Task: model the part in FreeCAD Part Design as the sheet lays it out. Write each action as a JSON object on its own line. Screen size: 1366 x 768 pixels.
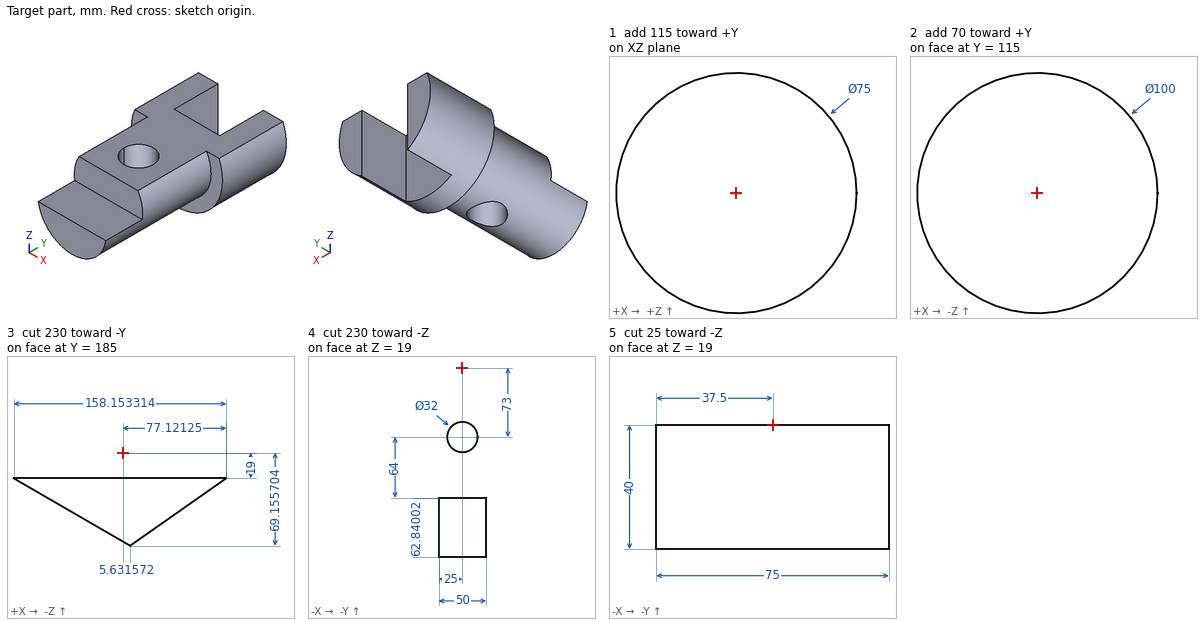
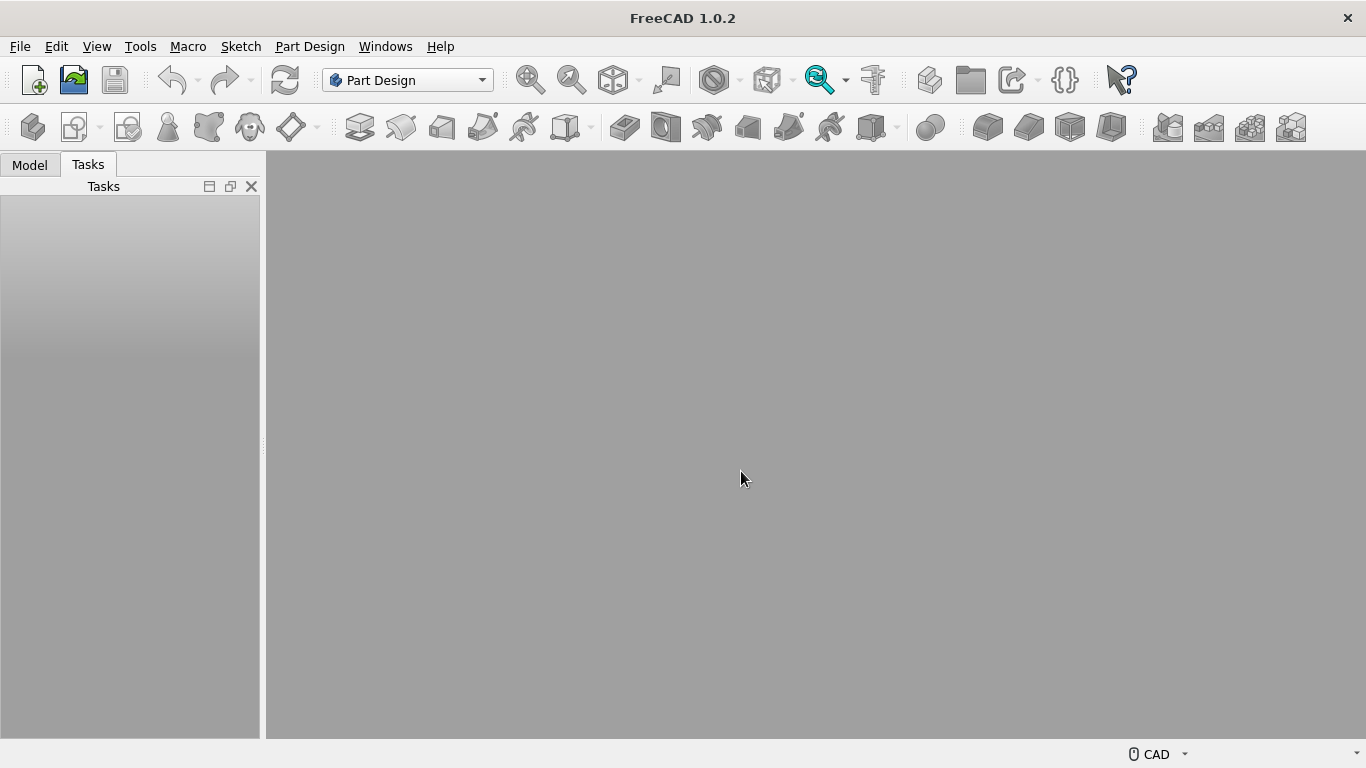
{"action": "left_click", "coordinate": [33, 80]}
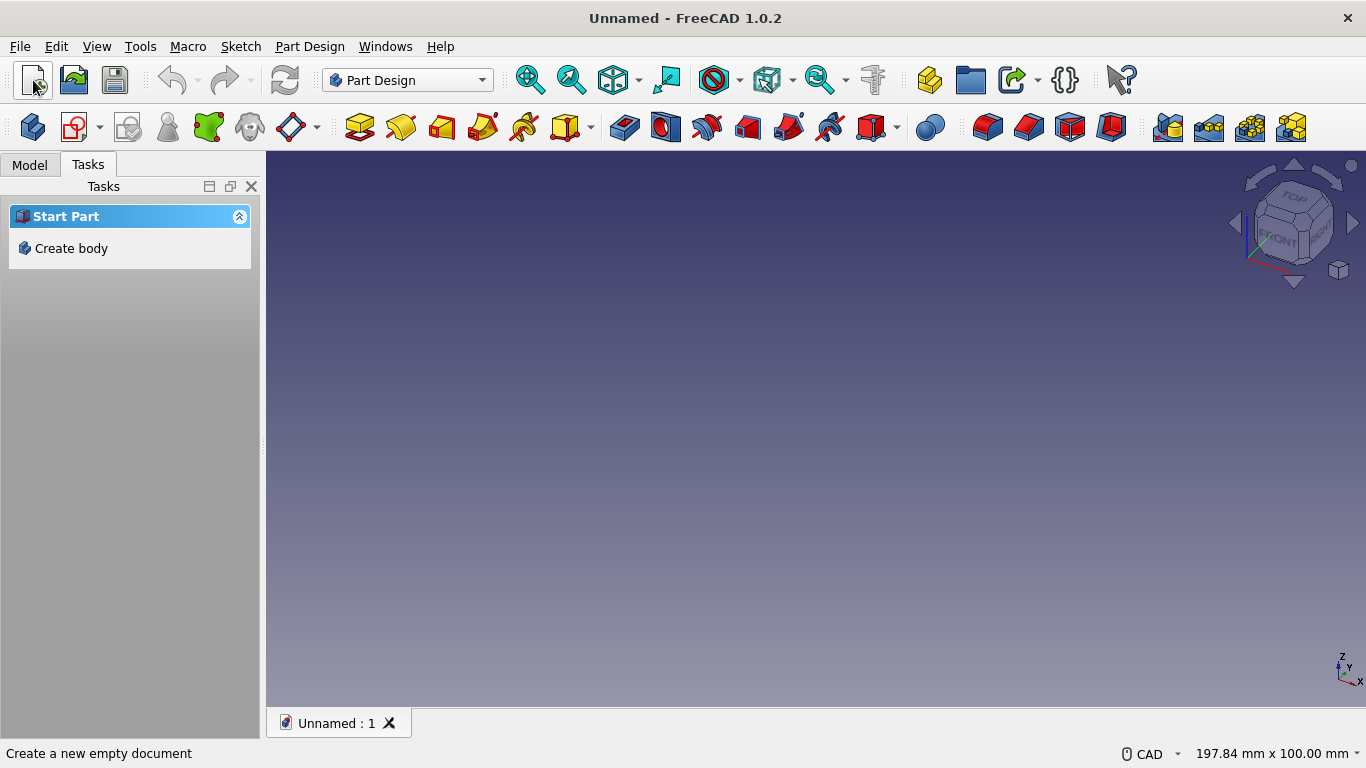
{"action": "left_click", "coordinate": [74, 128]}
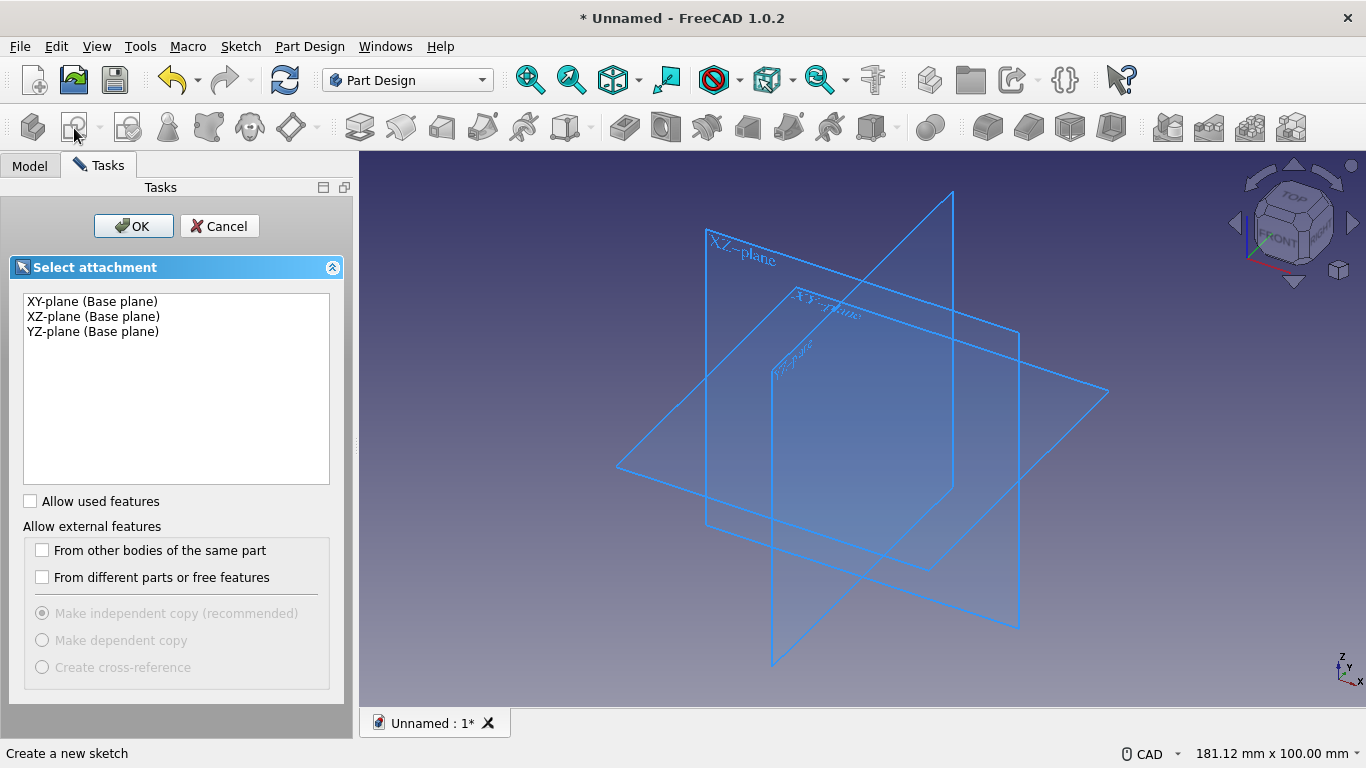
{"action": "left_click", "coordinate": [84, 316]}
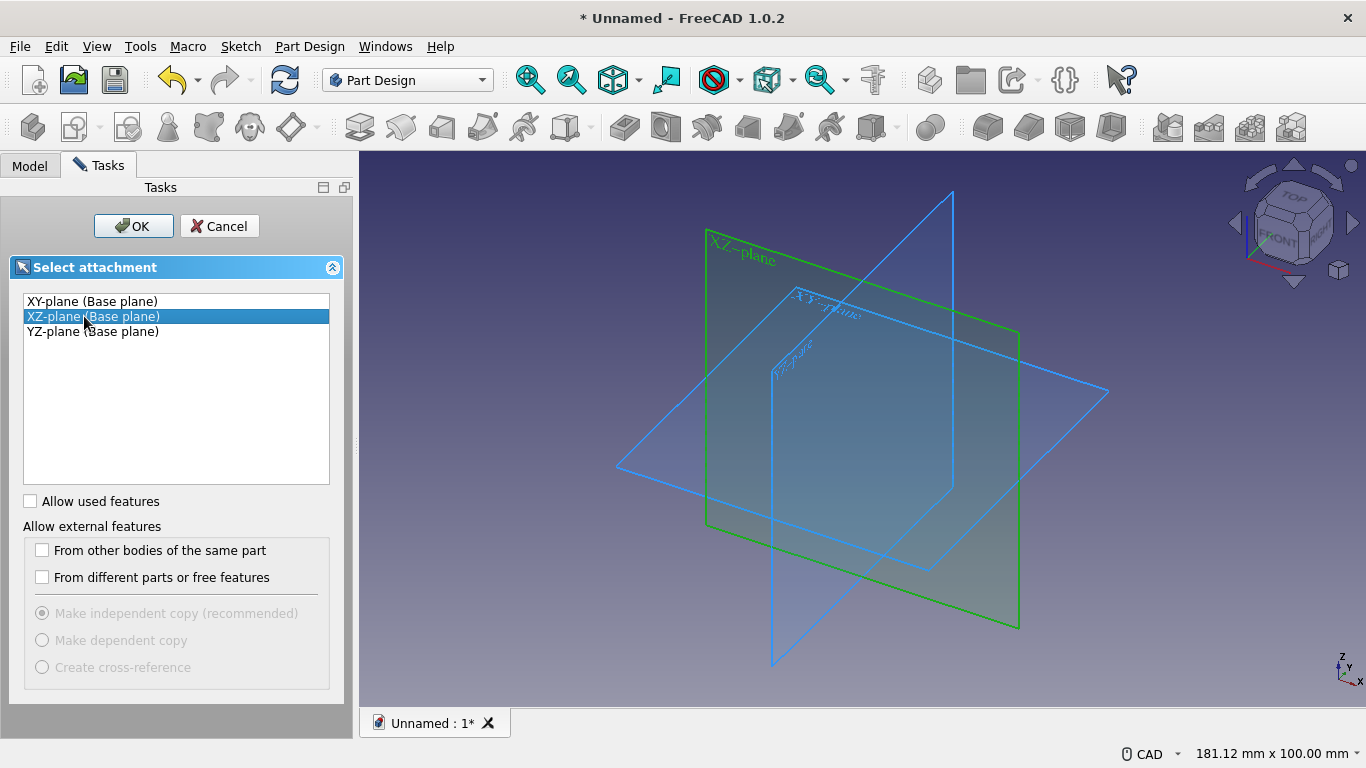
{"action": "left_click", "coordinate": [134, 226]}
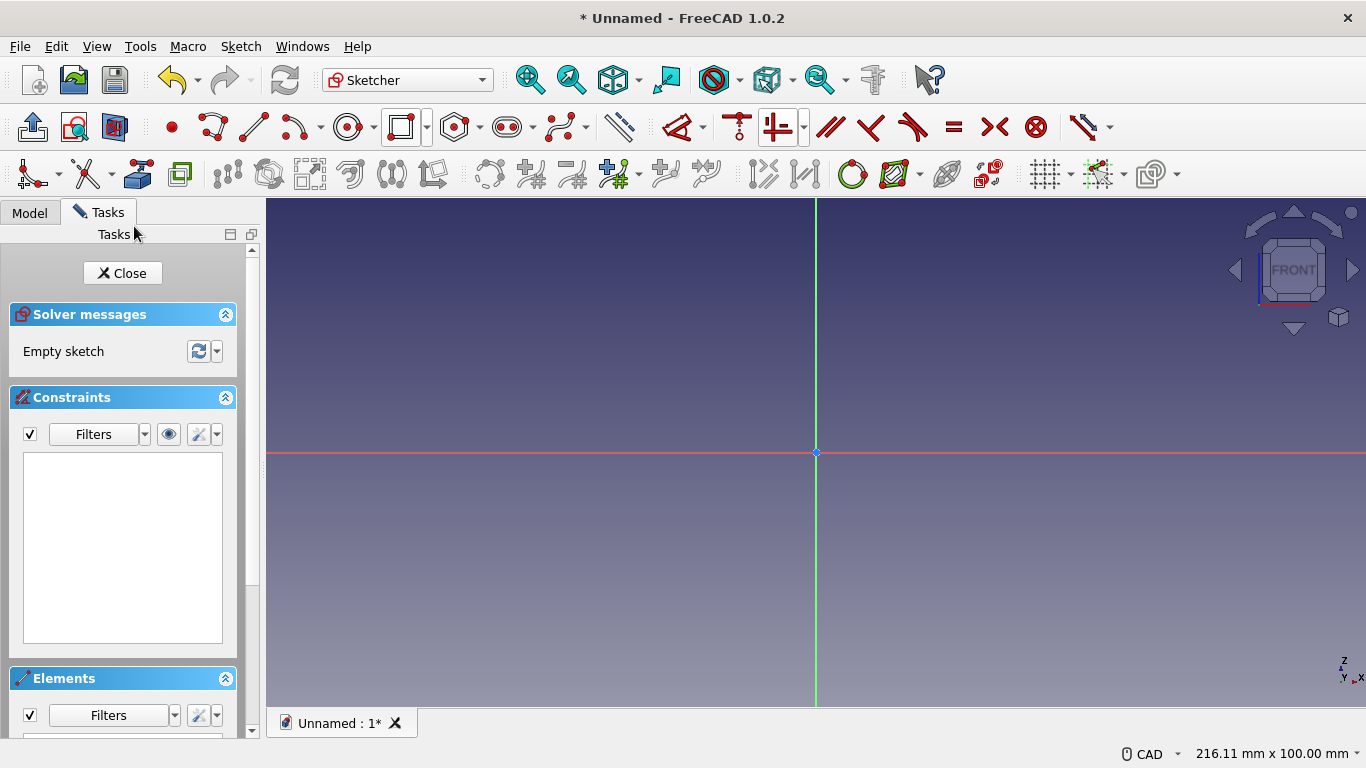
{"action": "left_click", "coordinate": [348, 128]}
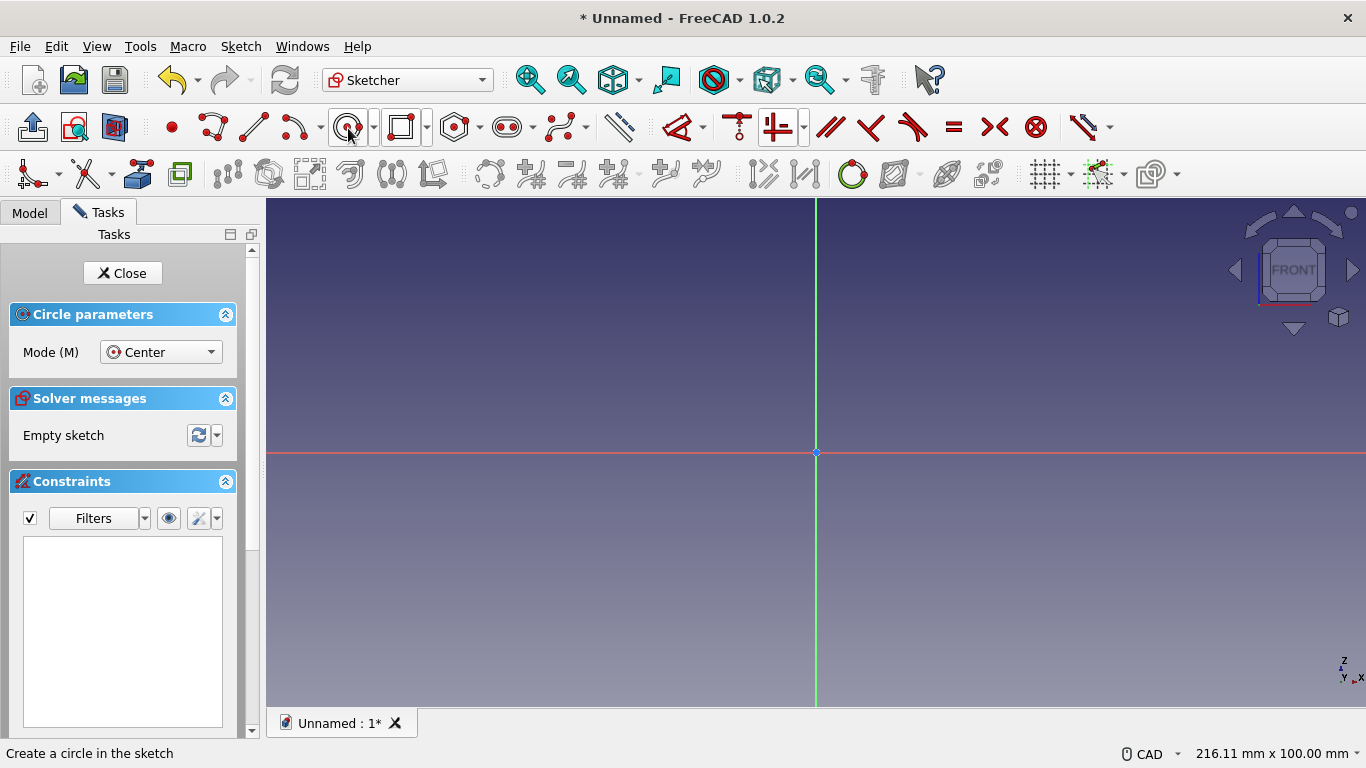
{"action": "left_click", "coordinate": [816, 452]}
{"action": "left_click", "coordinate": [951, 318]}
{"action": "key", "text": "Escape"}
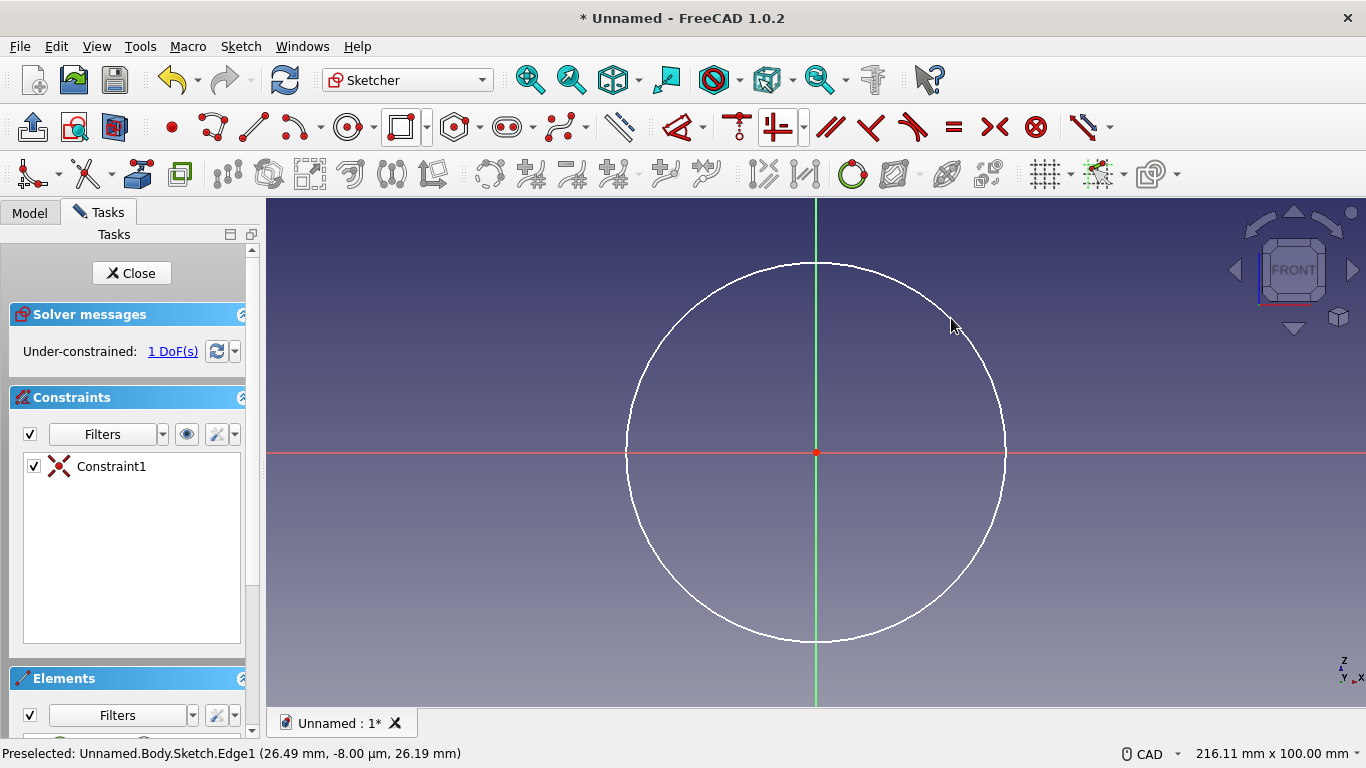
{"action": "left_click", "coordinate": [950, 318]}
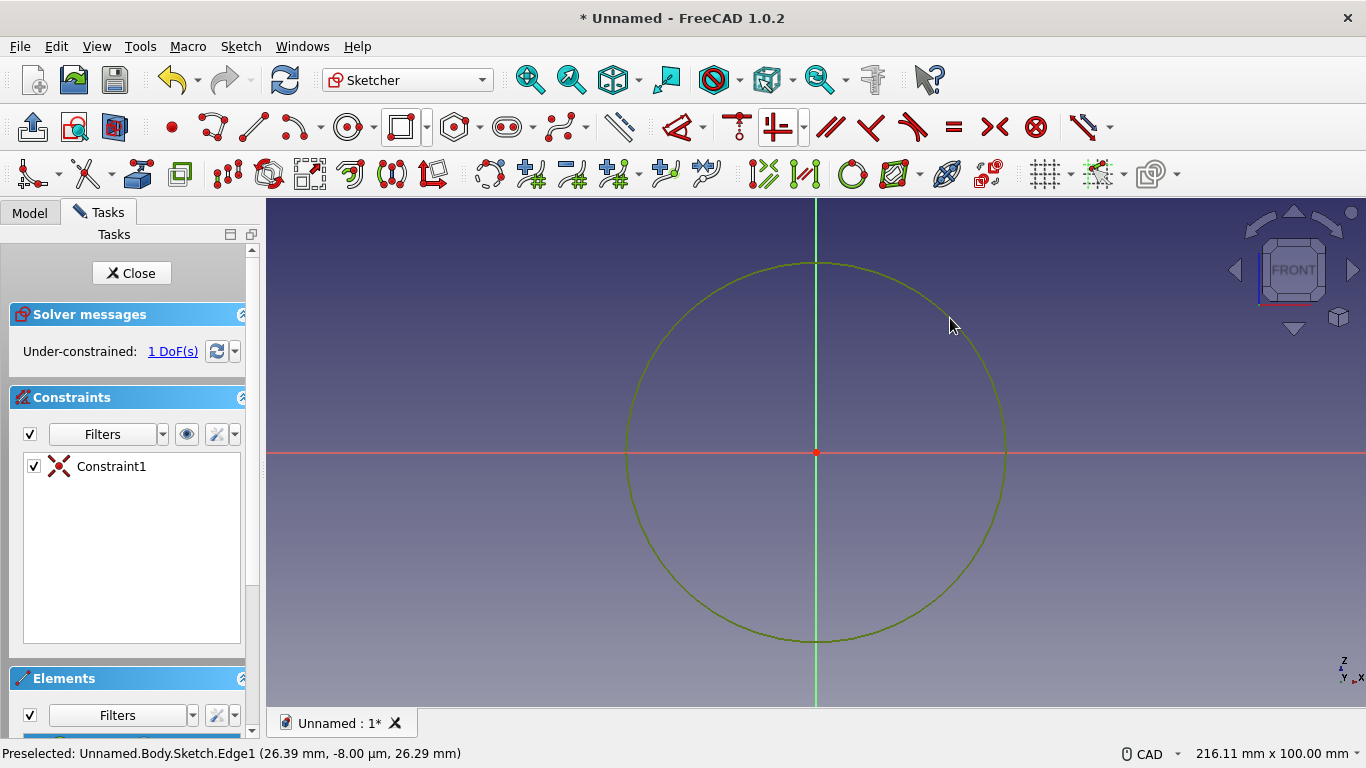
{"action": "left_click", "coordinate": [702, 128]}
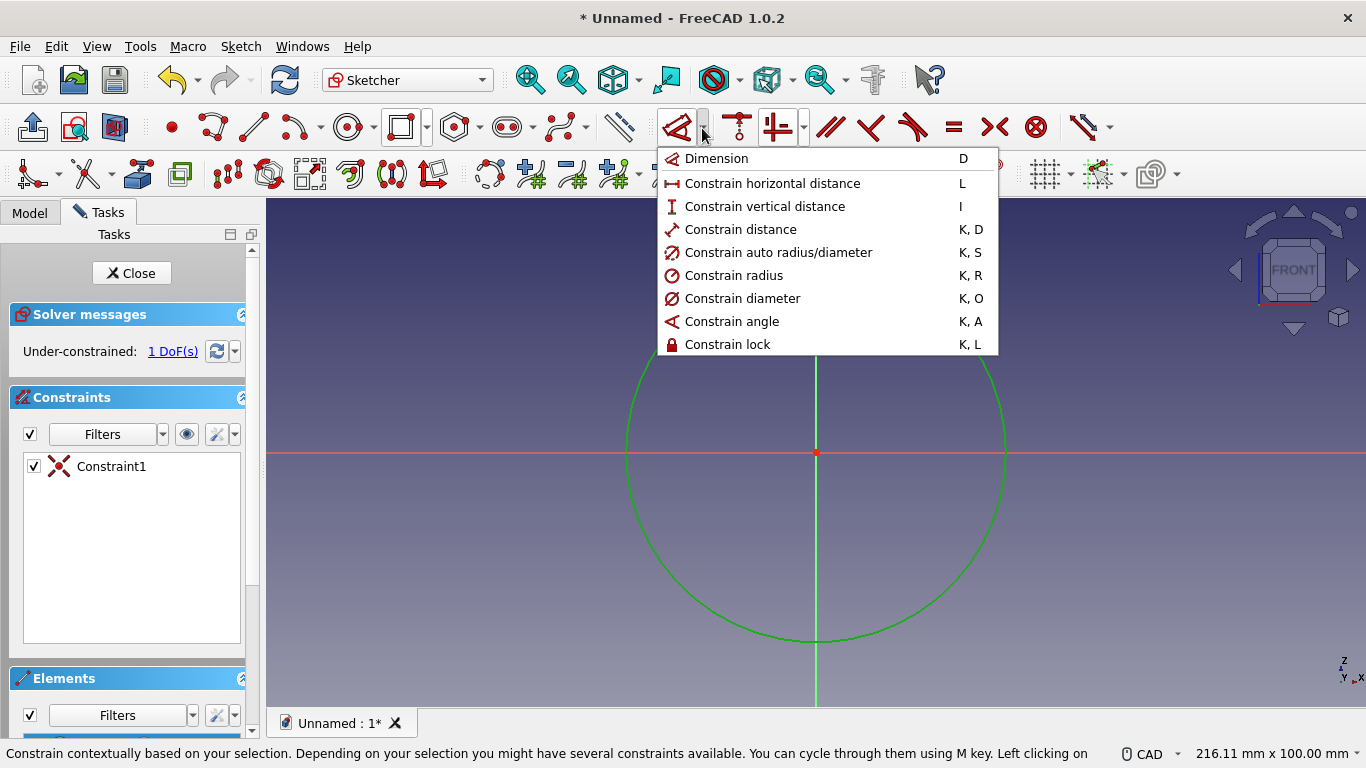
{"action": "left_click", "coordinate": [828, 298]}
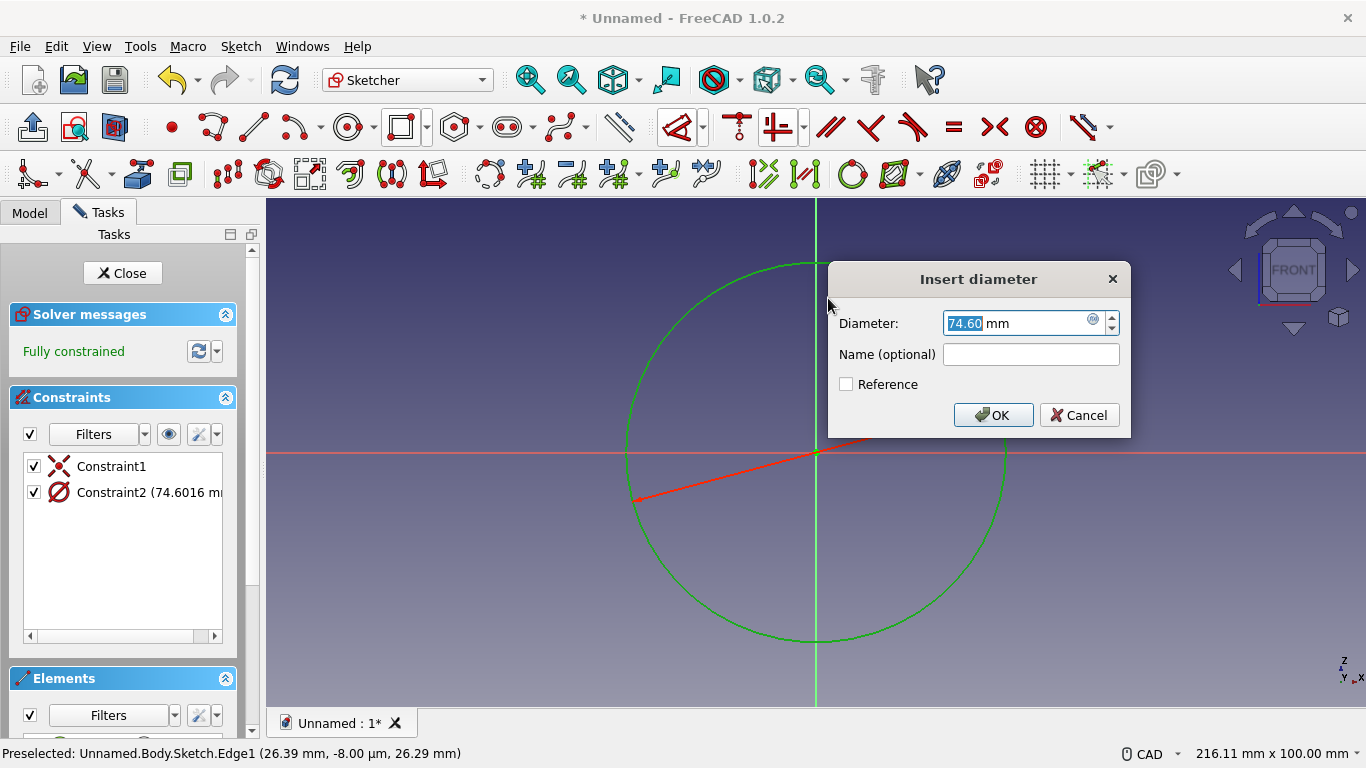
{"action": "type", "text": "75"}
{"action": "key", "text": "Return"}